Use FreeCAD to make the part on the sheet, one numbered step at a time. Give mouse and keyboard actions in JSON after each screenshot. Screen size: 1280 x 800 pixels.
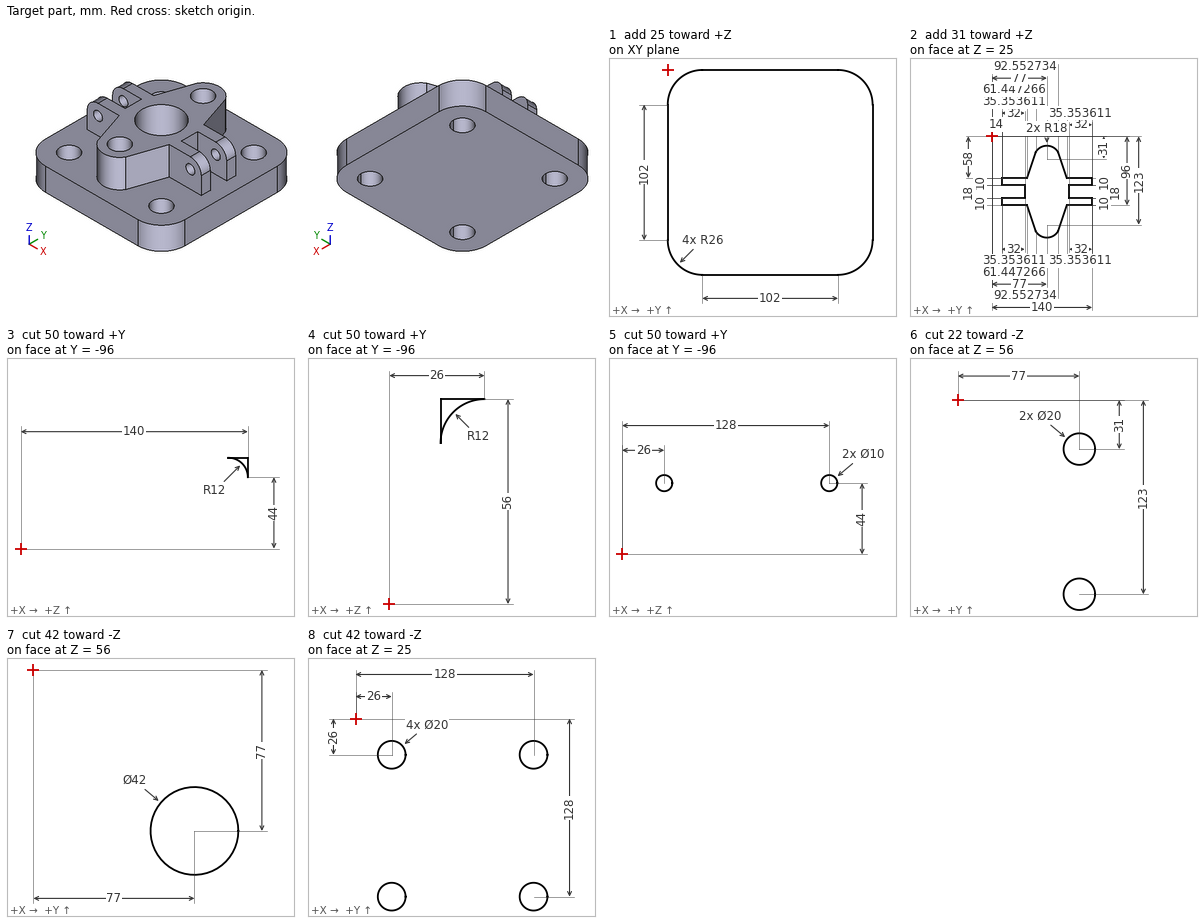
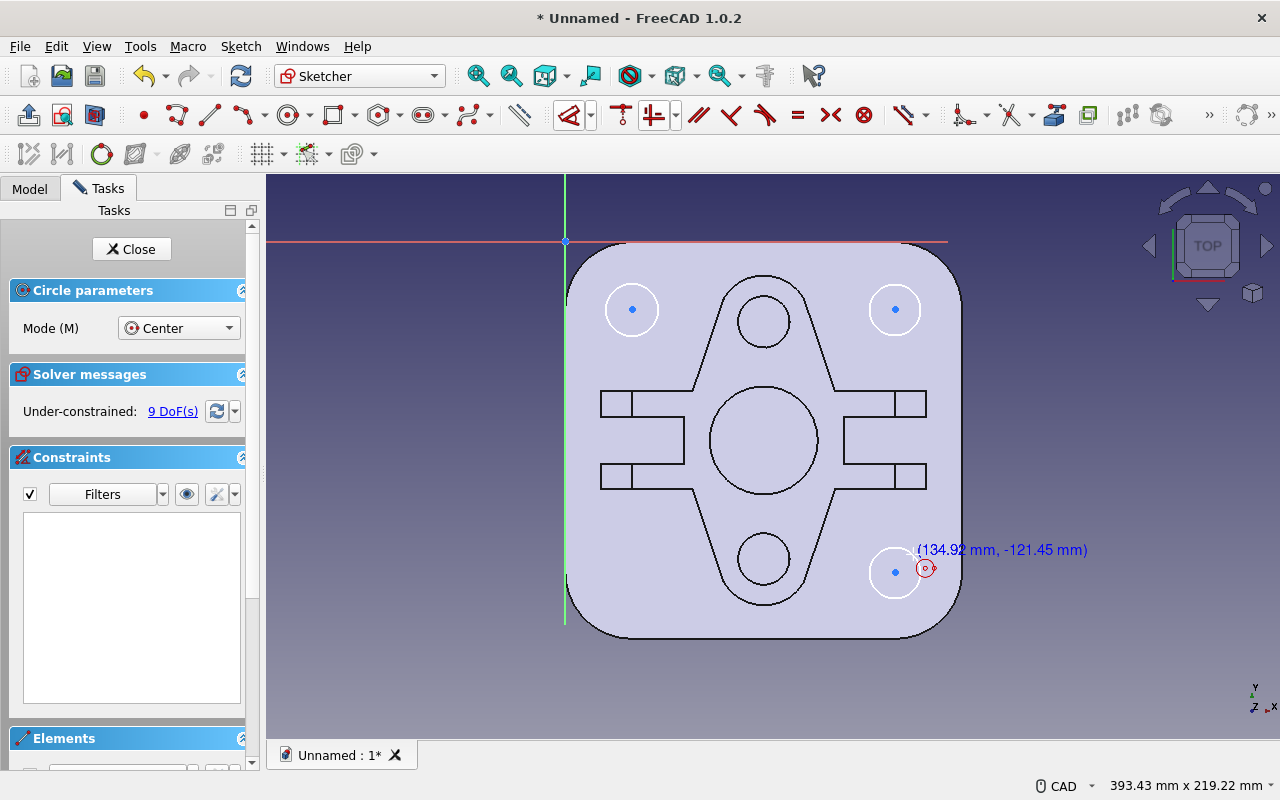
{"action": "left_click", "coordinate": [632, 572]}
{"action": "left_click", "coordinate": [651, 554]}
{"action": "key", "text": "Escape"}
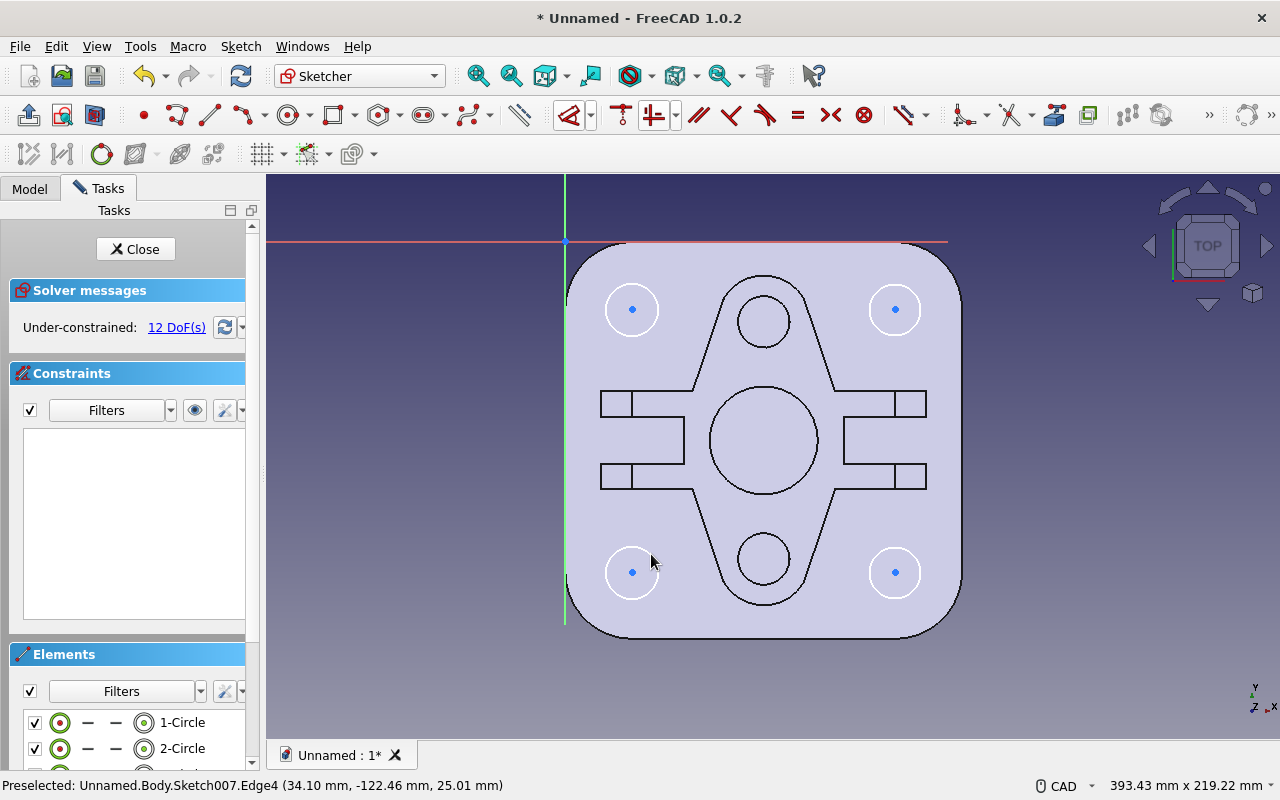
{"action": "left_click", "coordinate": [650, 291]}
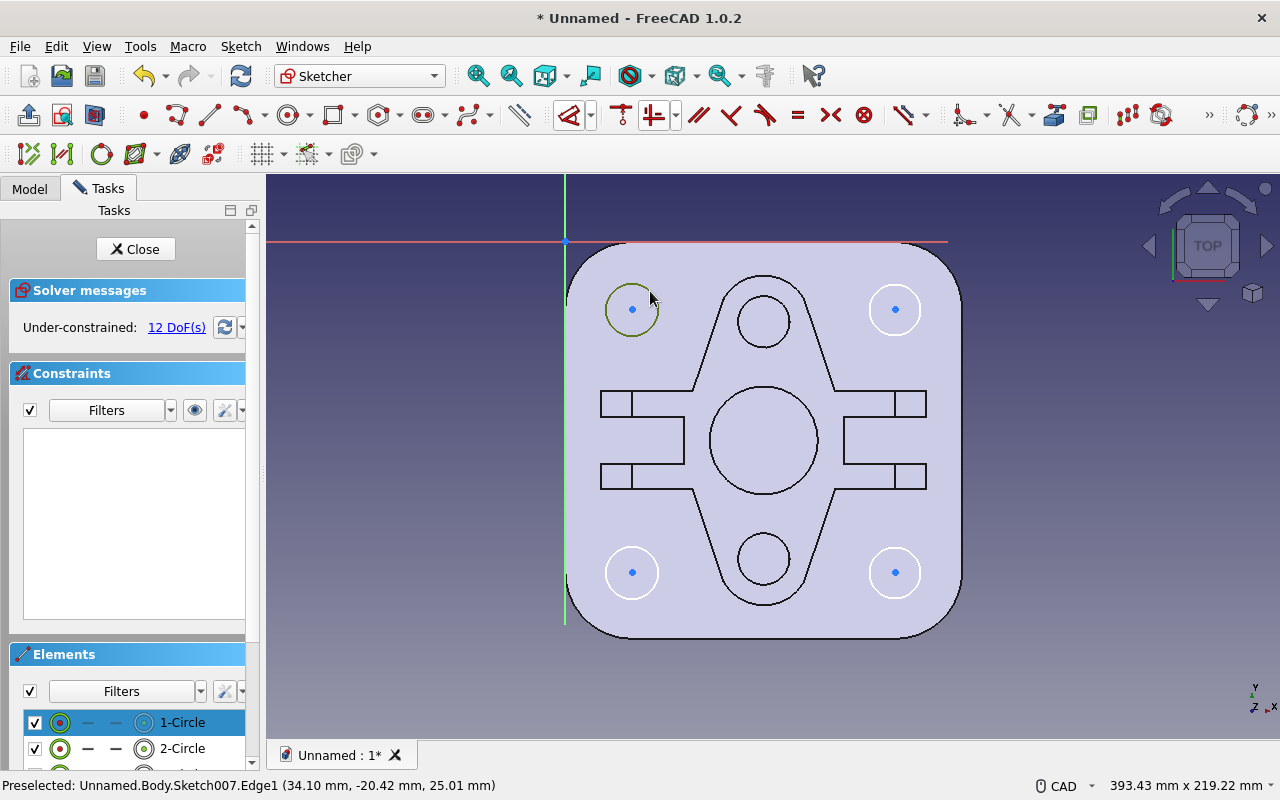
{"action": "left_click", "coordinate": [913, 292]}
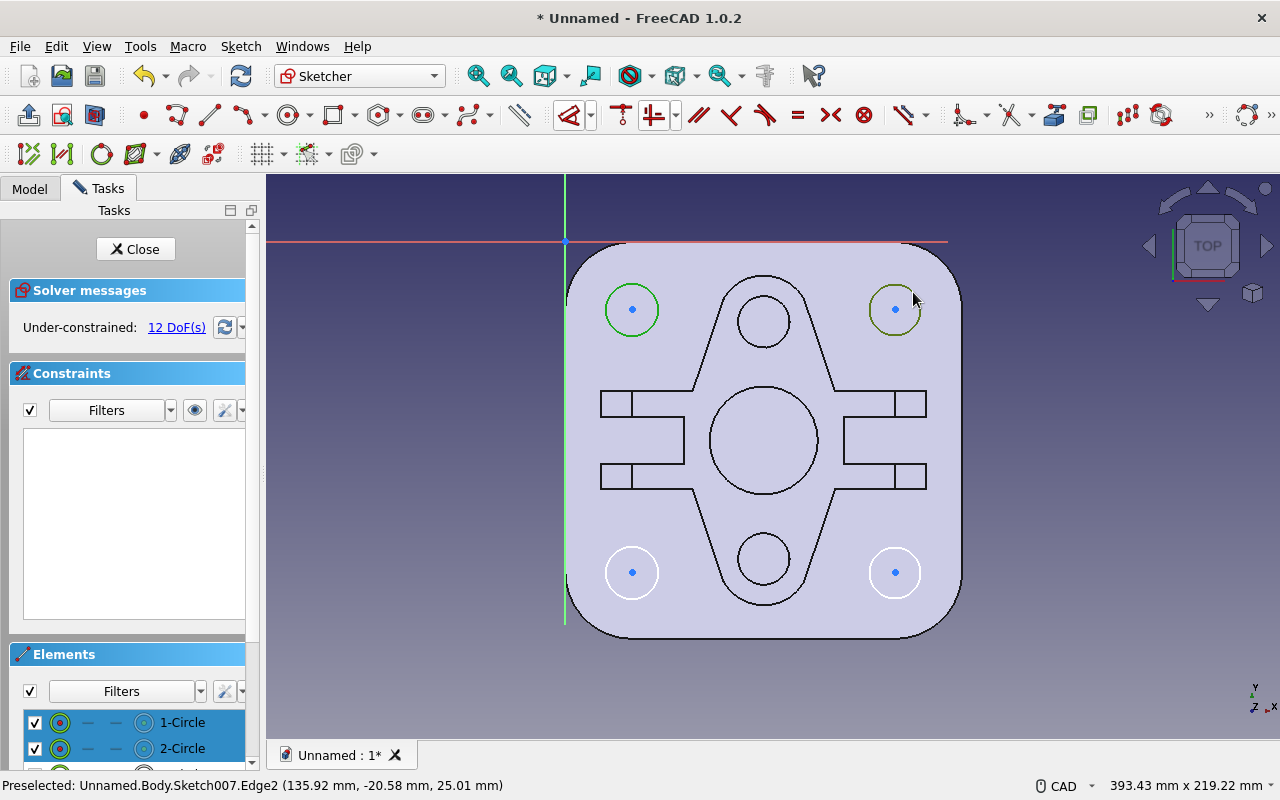
{"action": "left_click", "coordinate": [913, 555]}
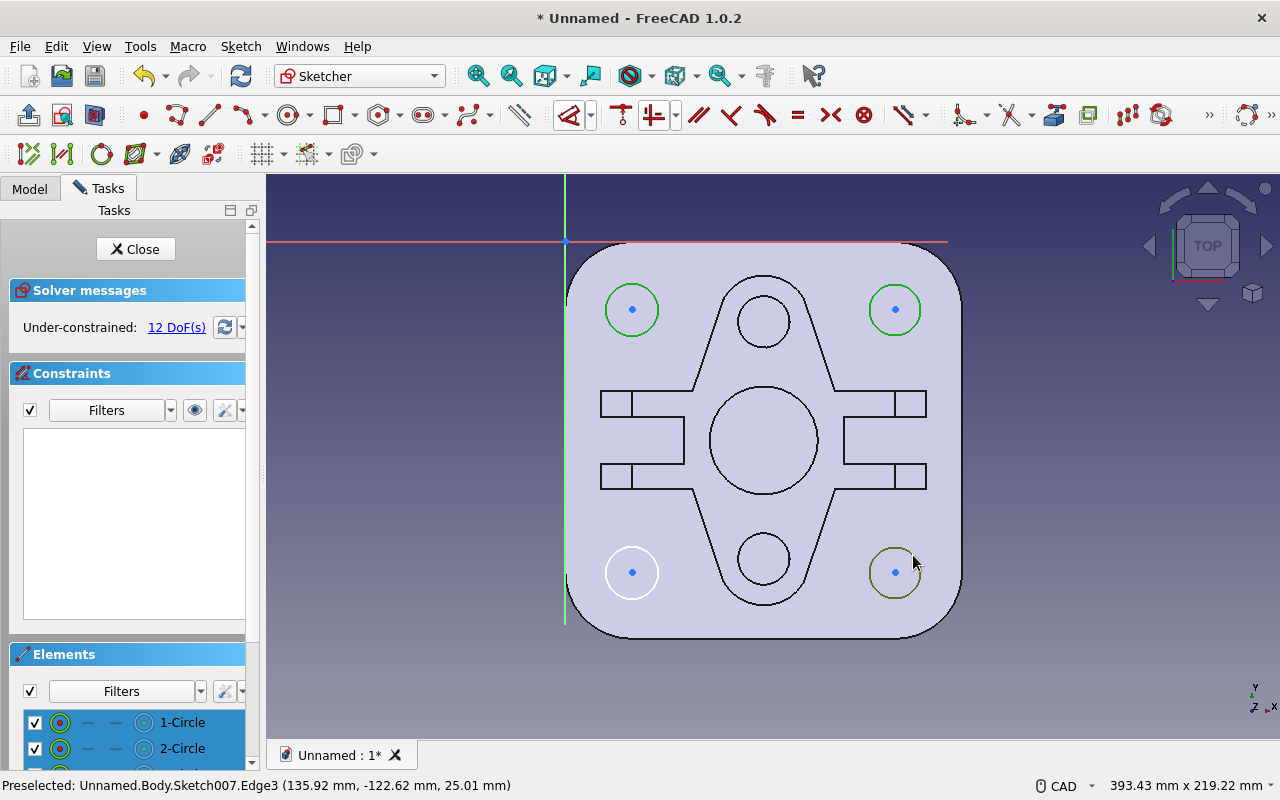
{"action": "left_click", "coordinate": [650, 554]}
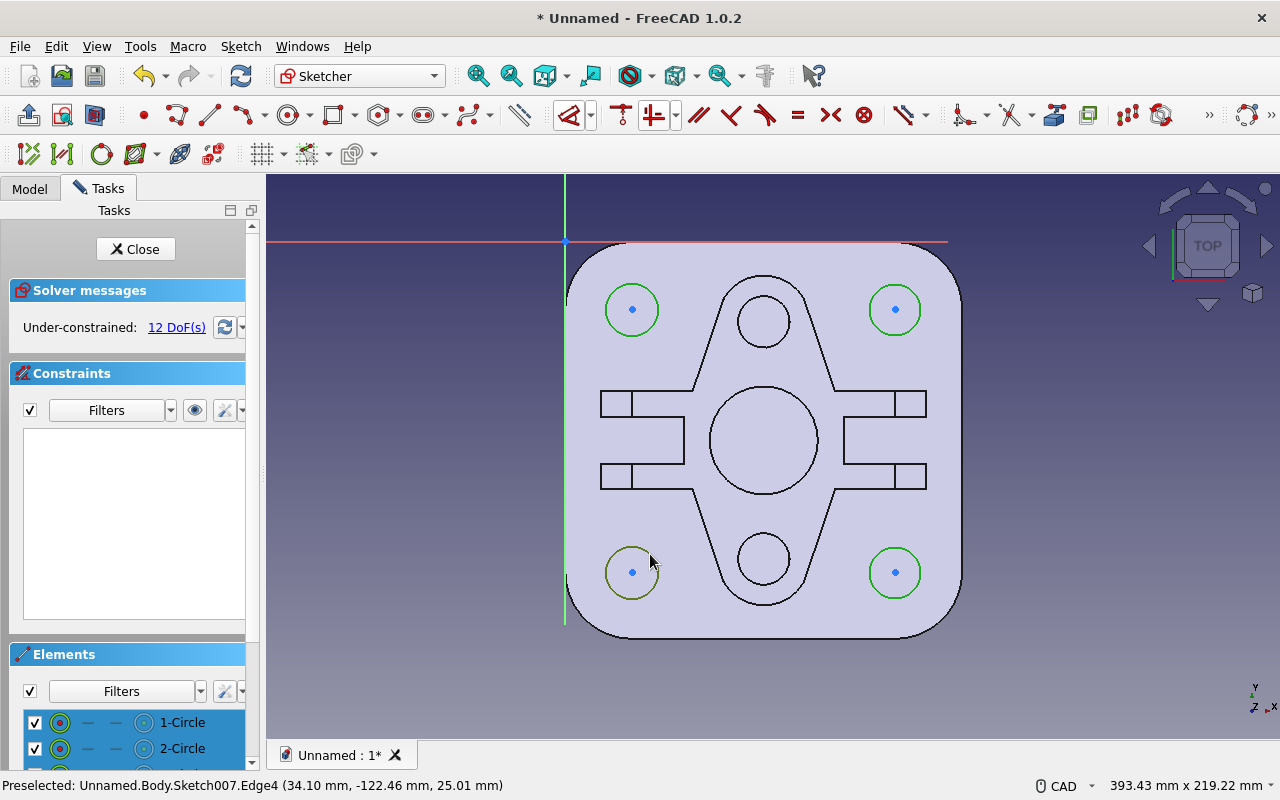
{"action": "left_click", "coordinate": [798, 116]}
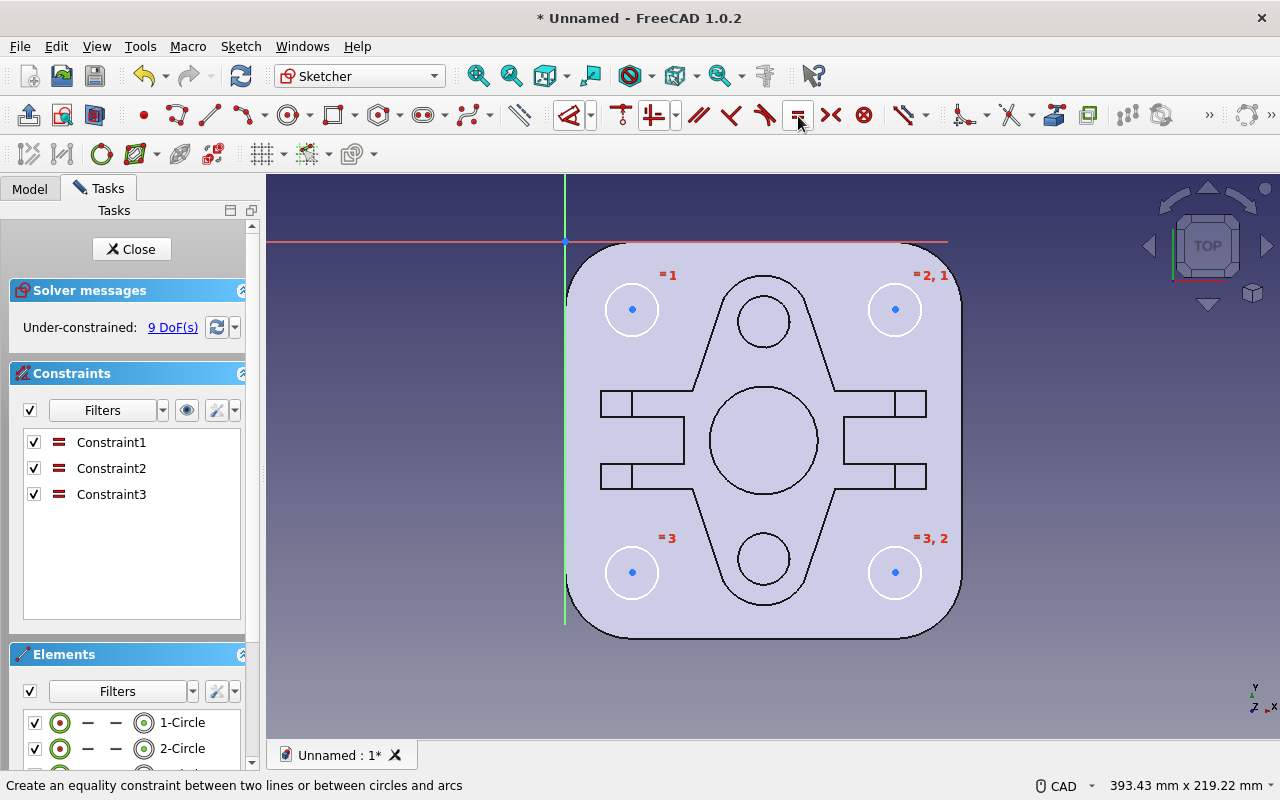
{"action": "left_click", "coordinate": [632, 310]}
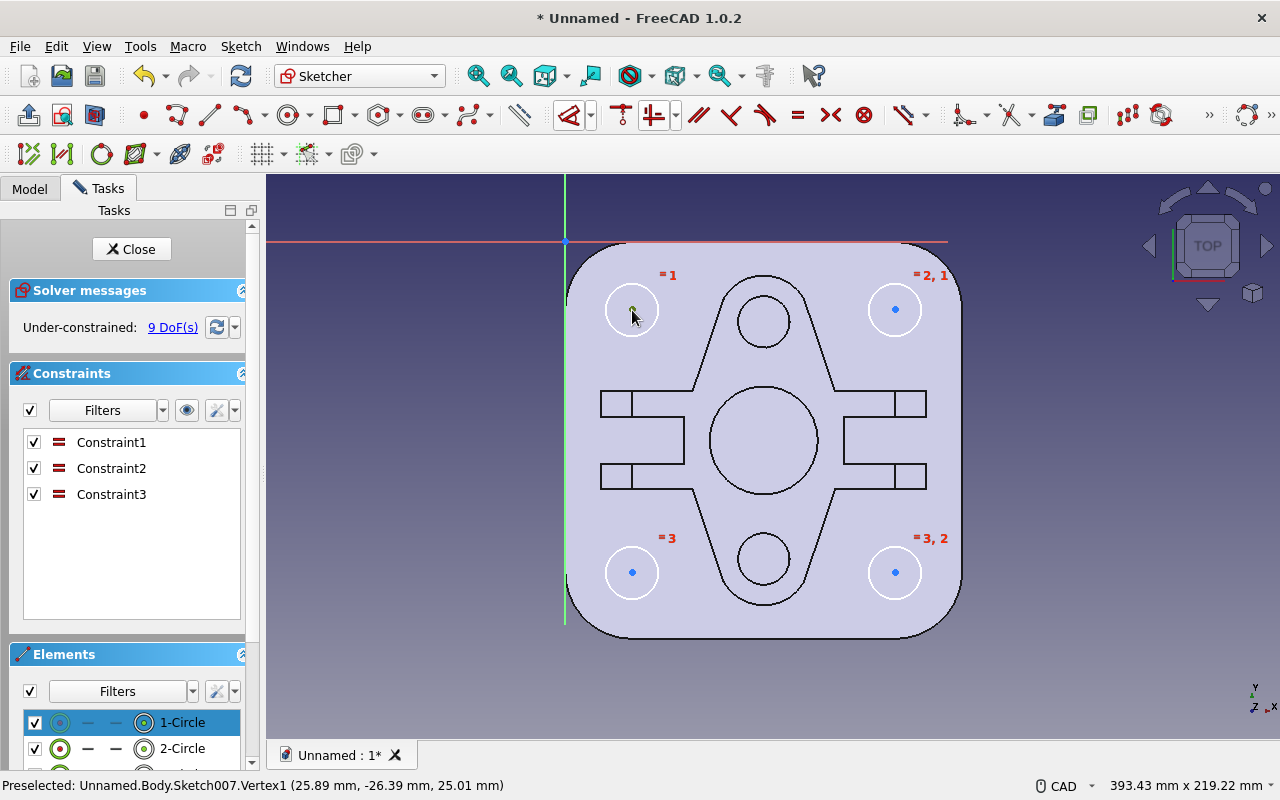
{"action": "left_click", "coordinate": [895, 310]}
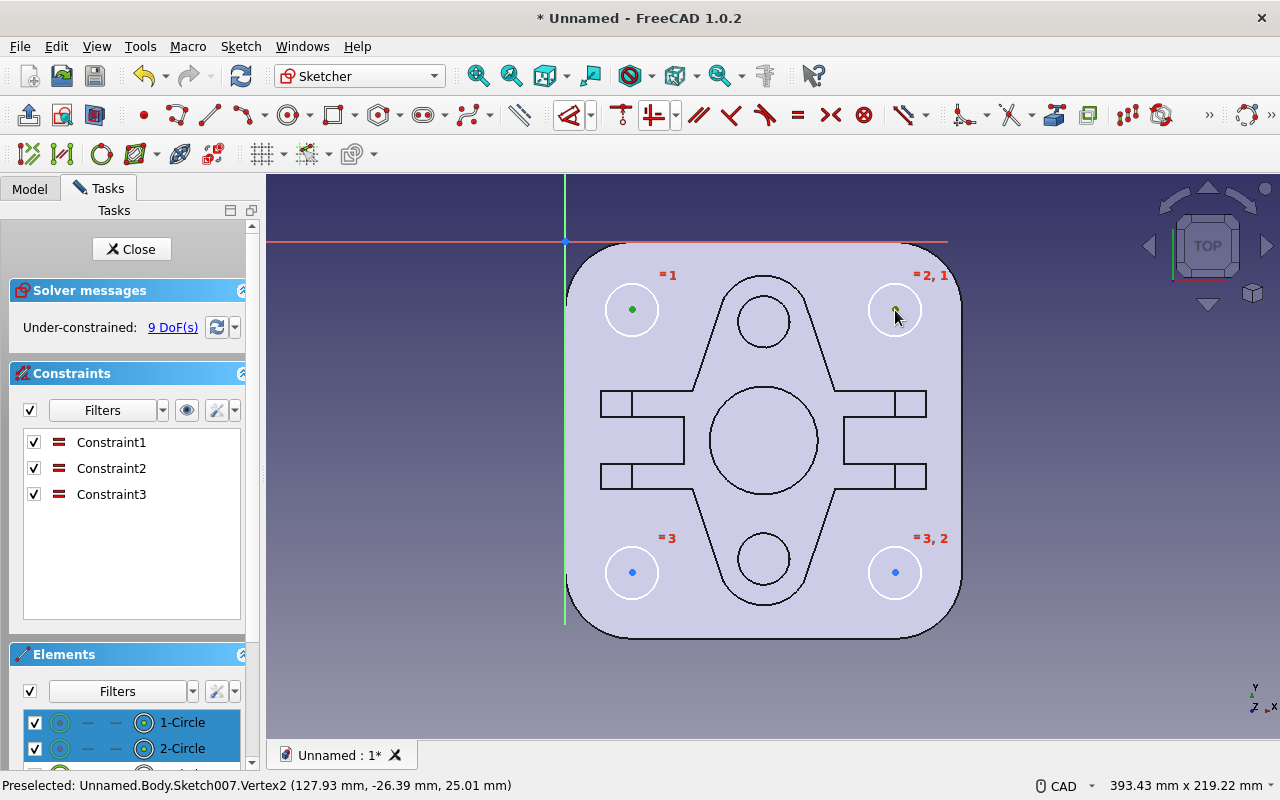
{"action": "left_click", "coordinate": [676, 116]}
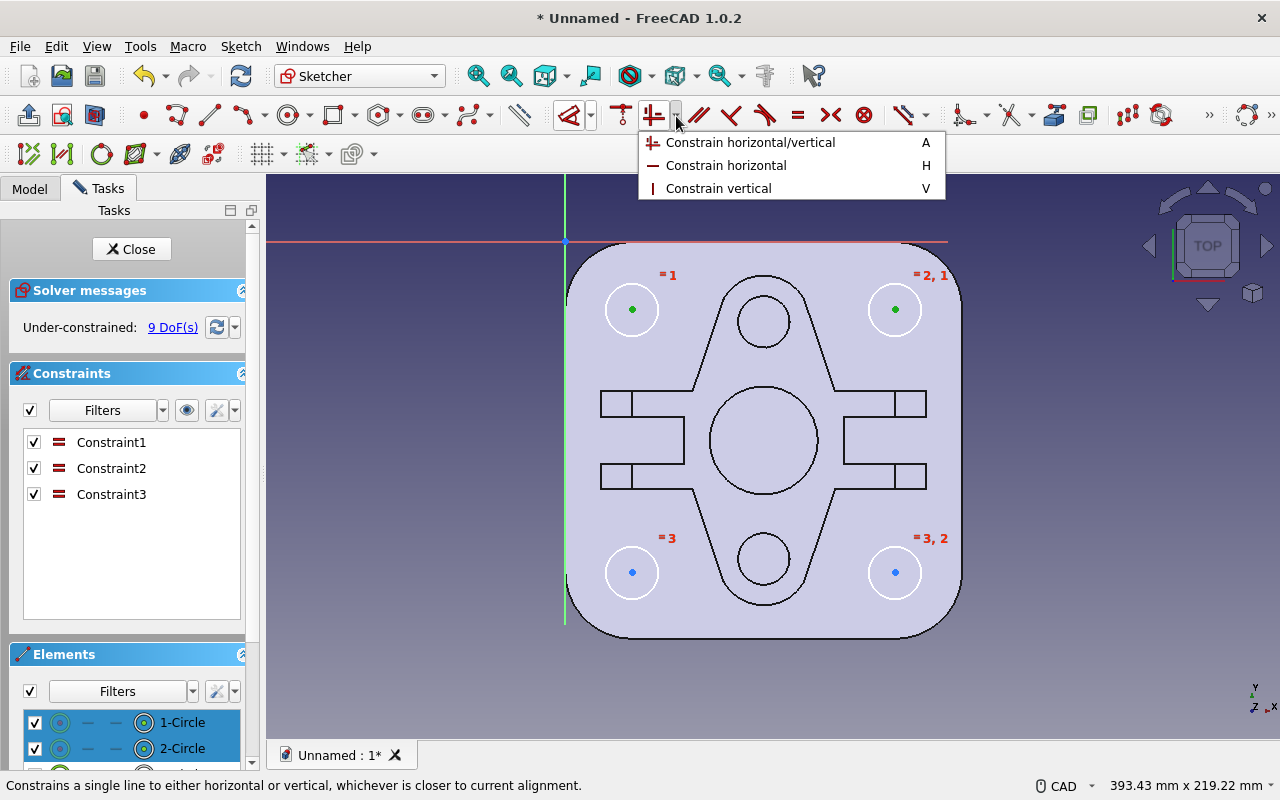
{"action": "left_click", "coordinate": [792, 166]}